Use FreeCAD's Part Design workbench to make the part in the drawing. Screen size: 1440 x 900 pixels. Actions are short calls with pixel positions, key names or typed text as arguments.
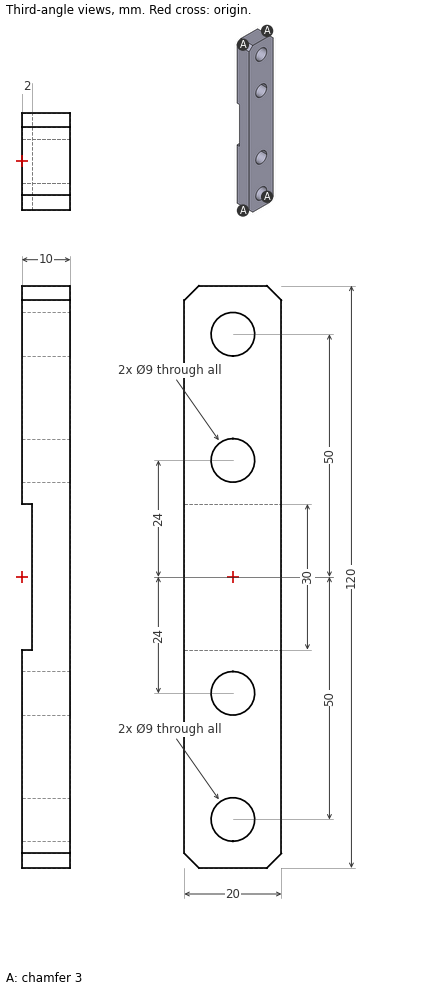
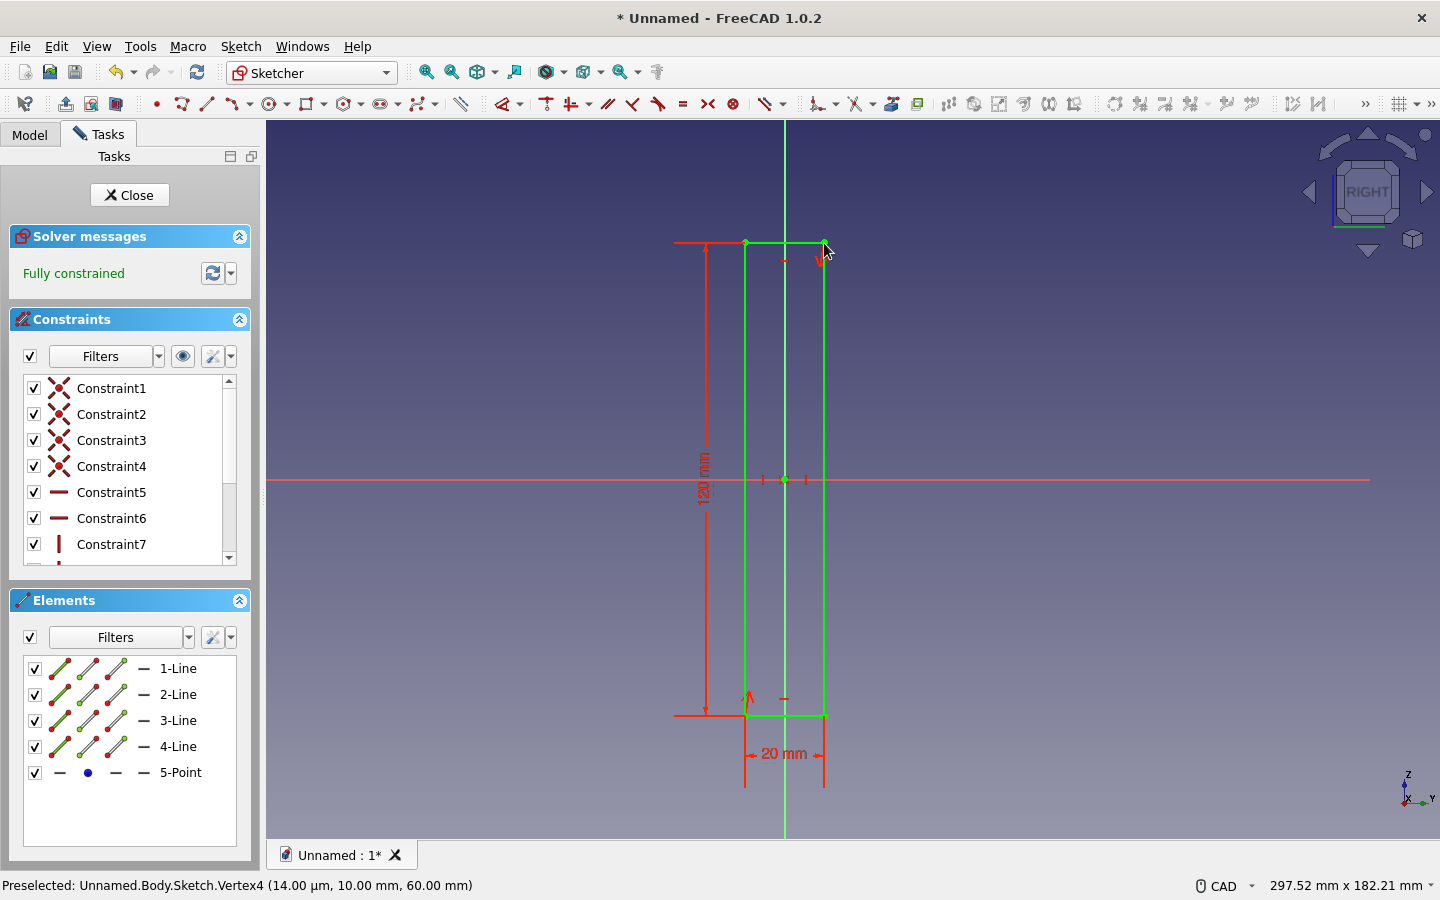
click(130, 195)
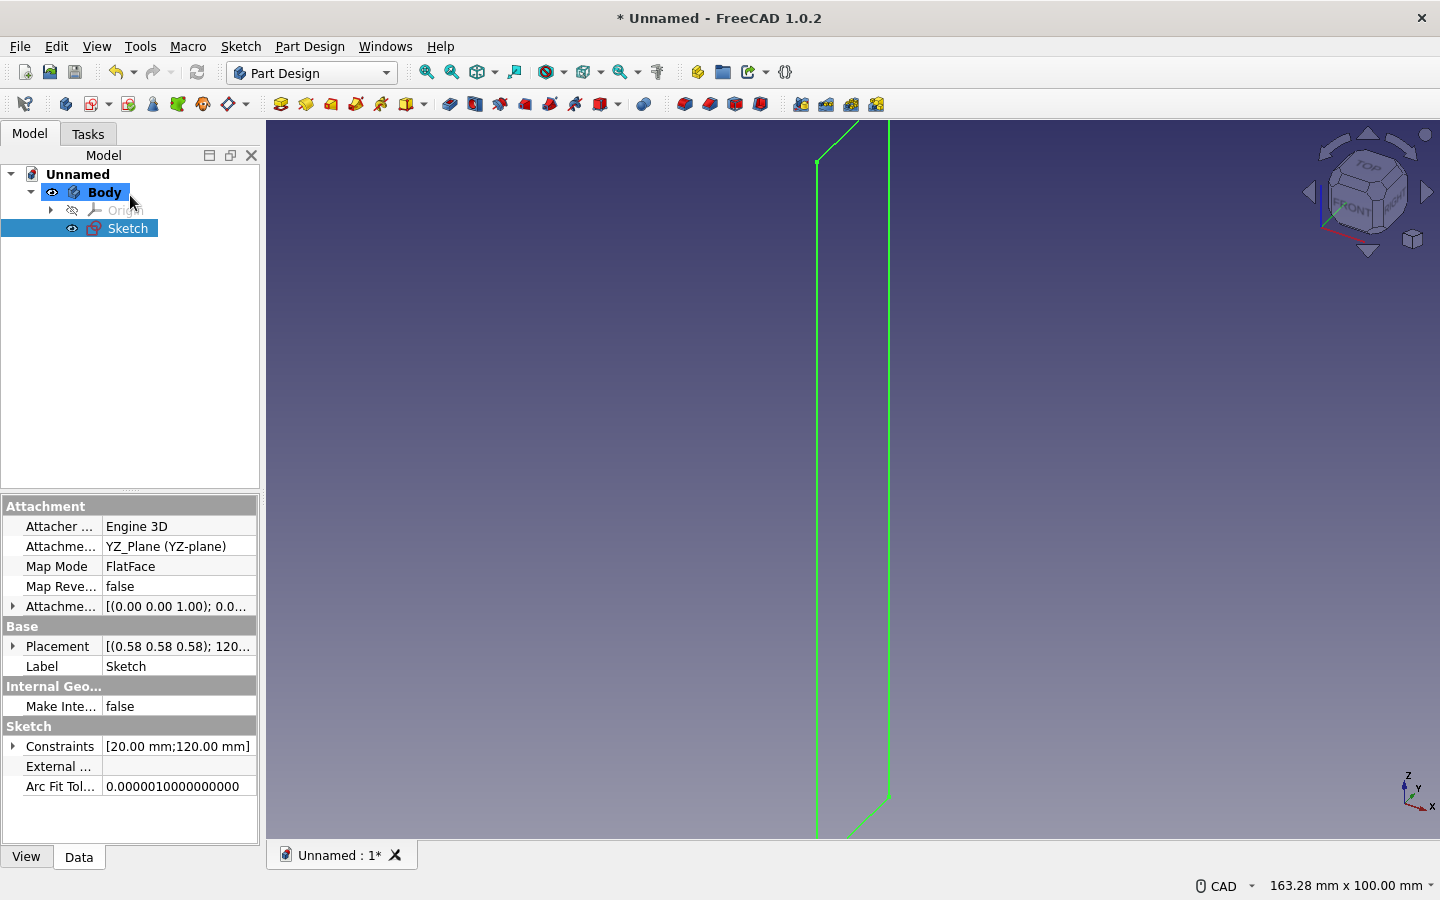
click(281, 104)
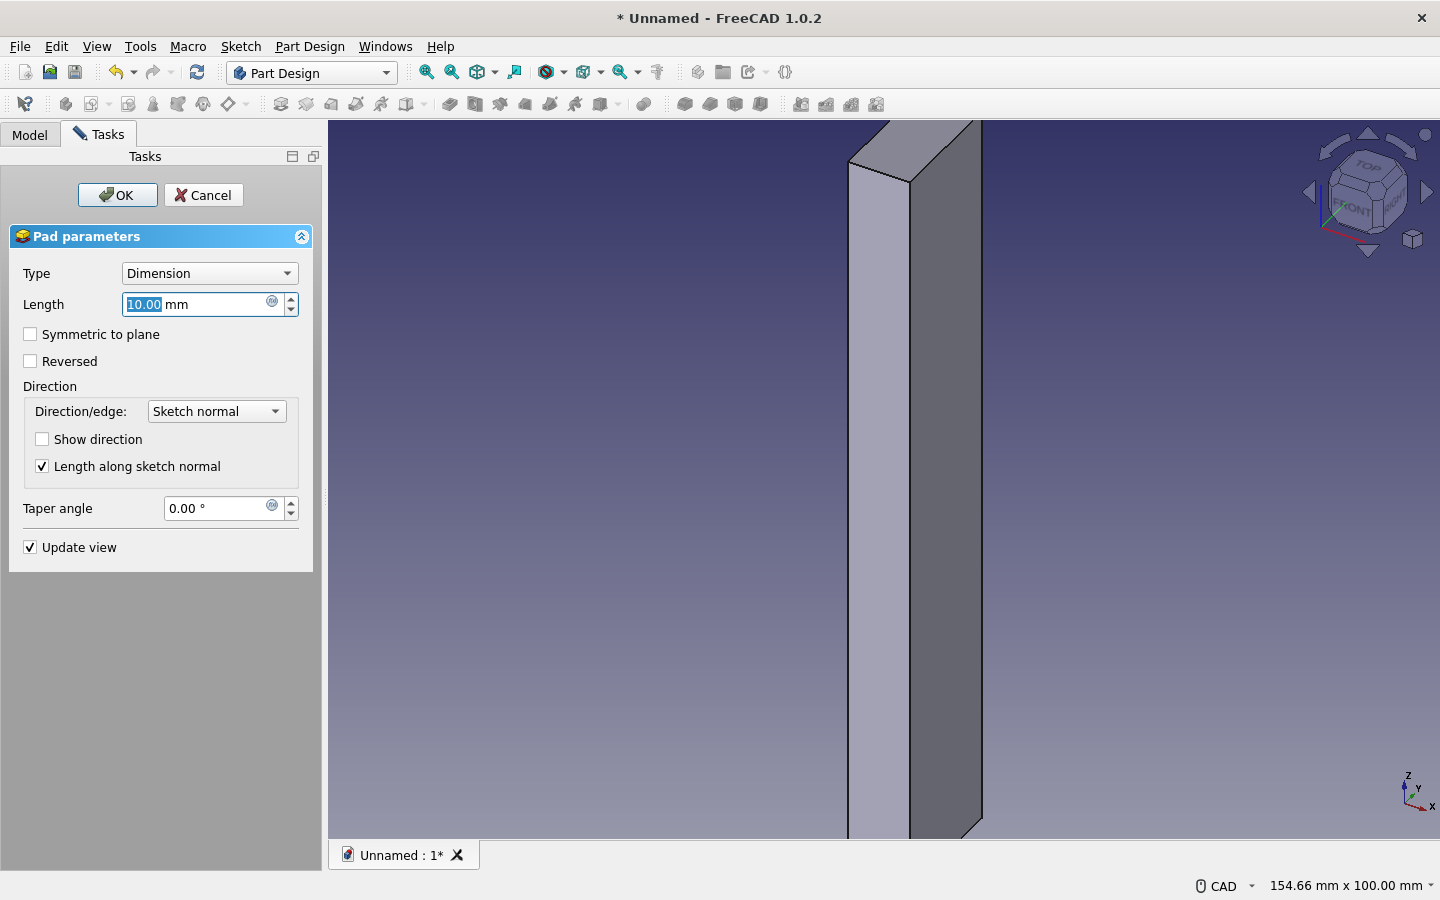
text(10)
key(Tab)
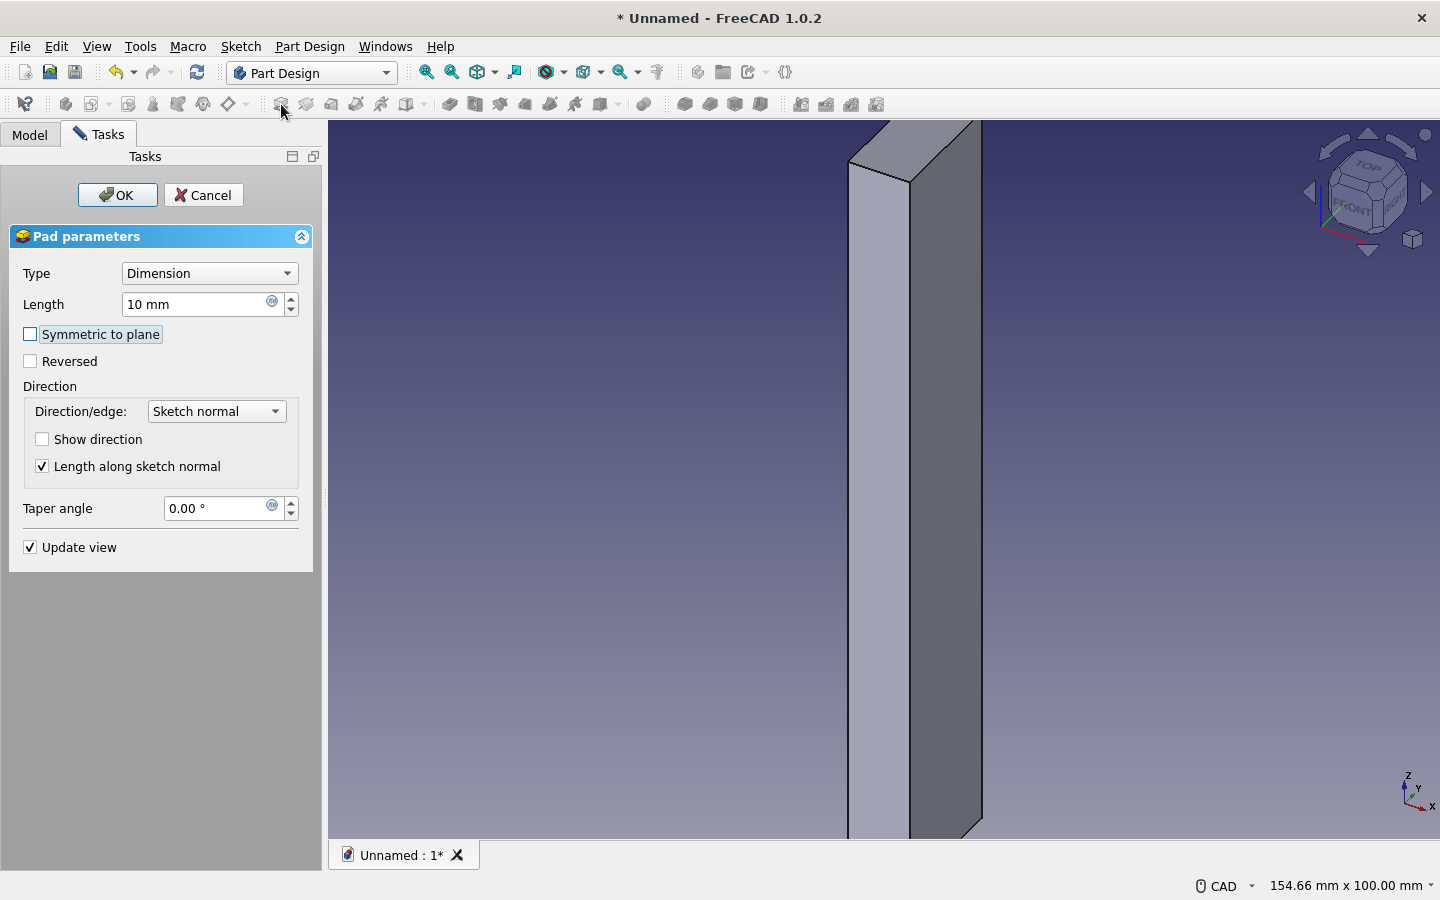
click(118, 195)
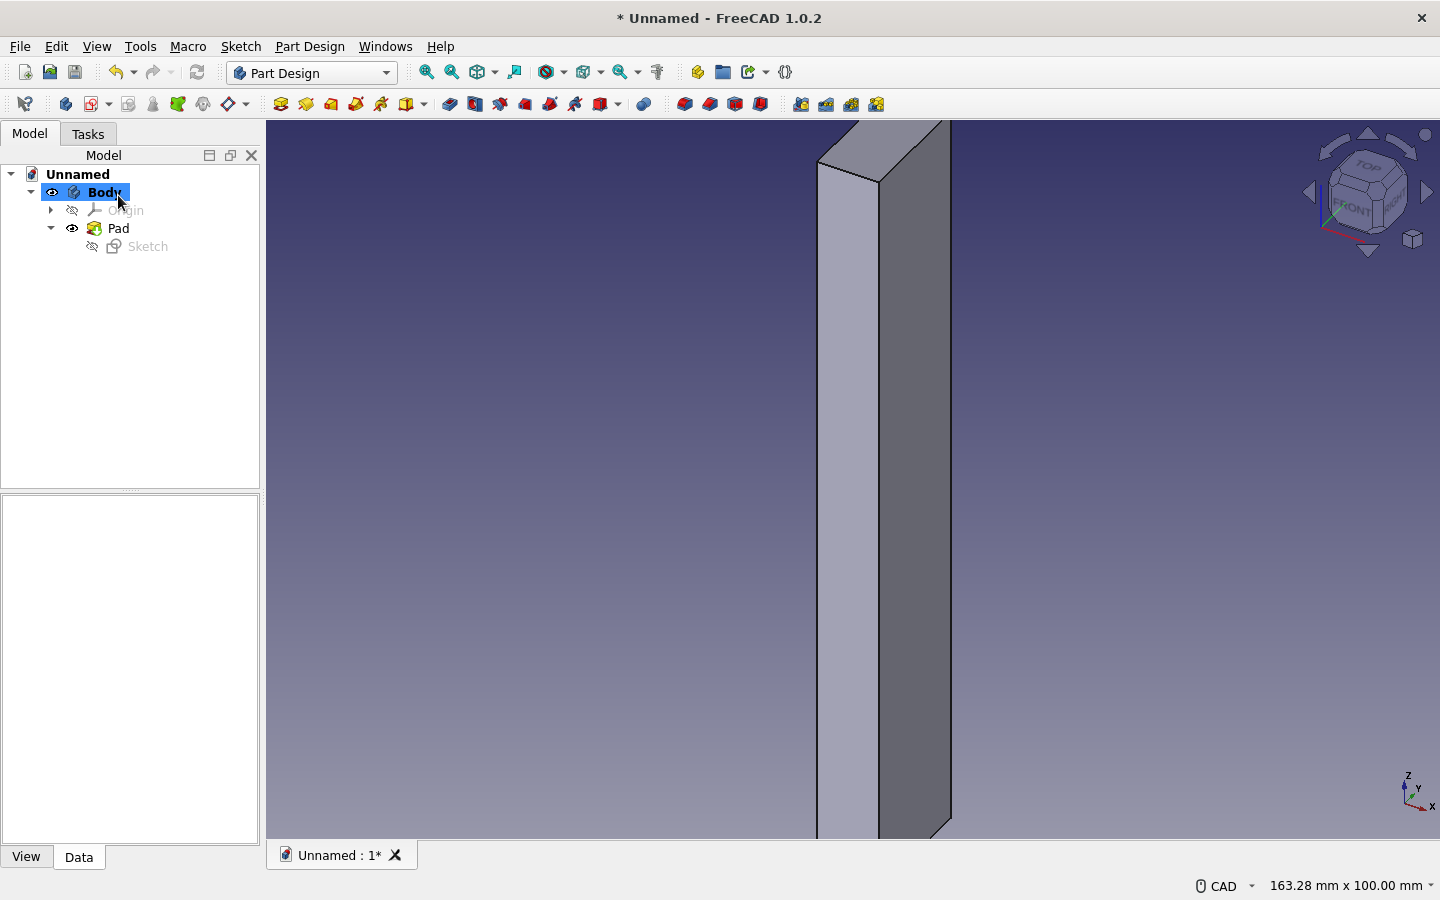
key(v)
key(f)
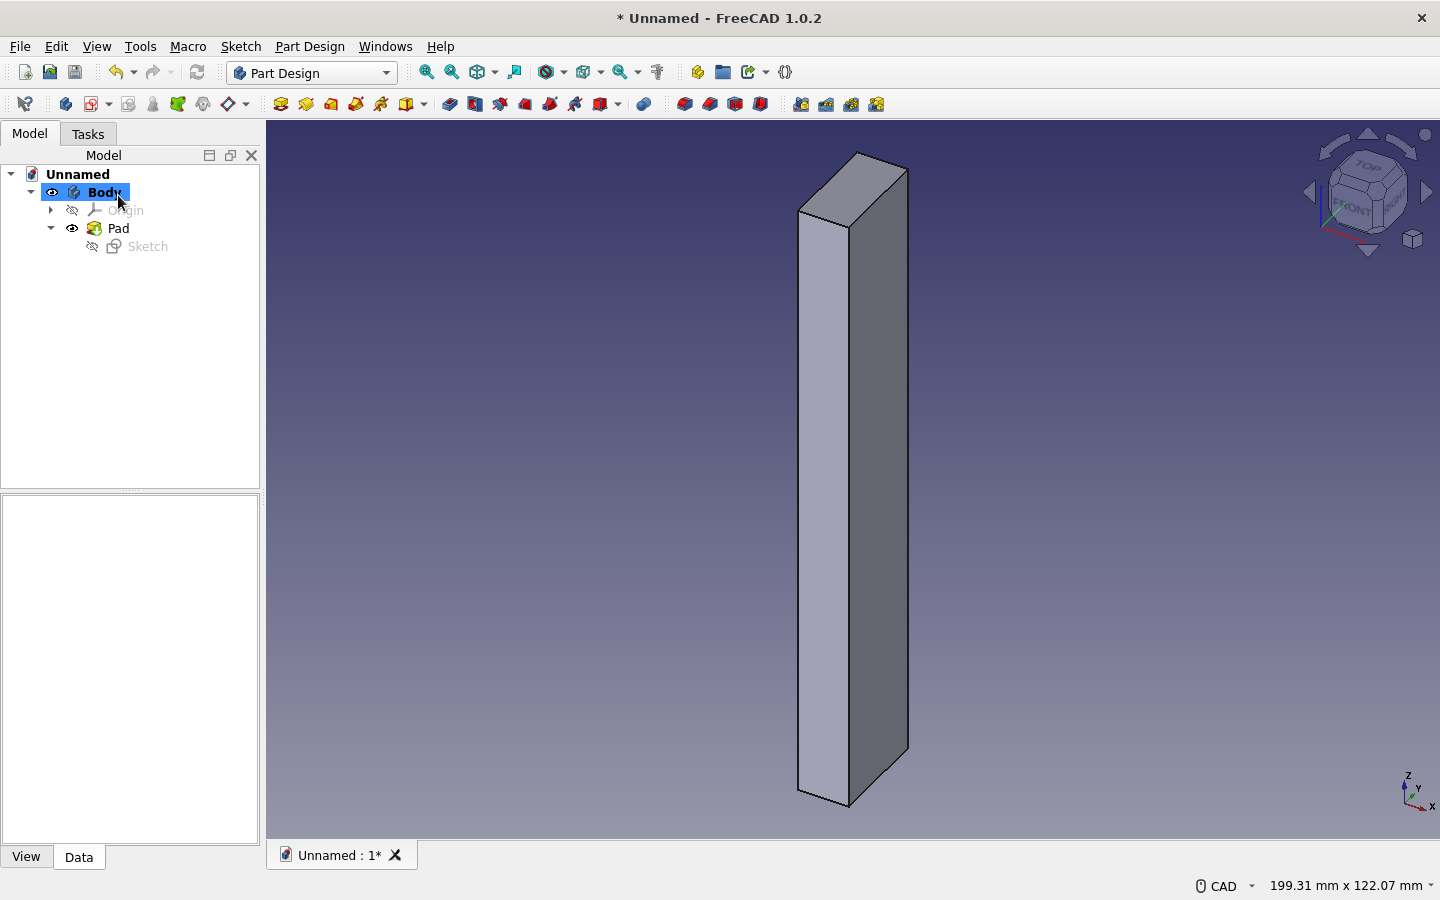
click(879, 652)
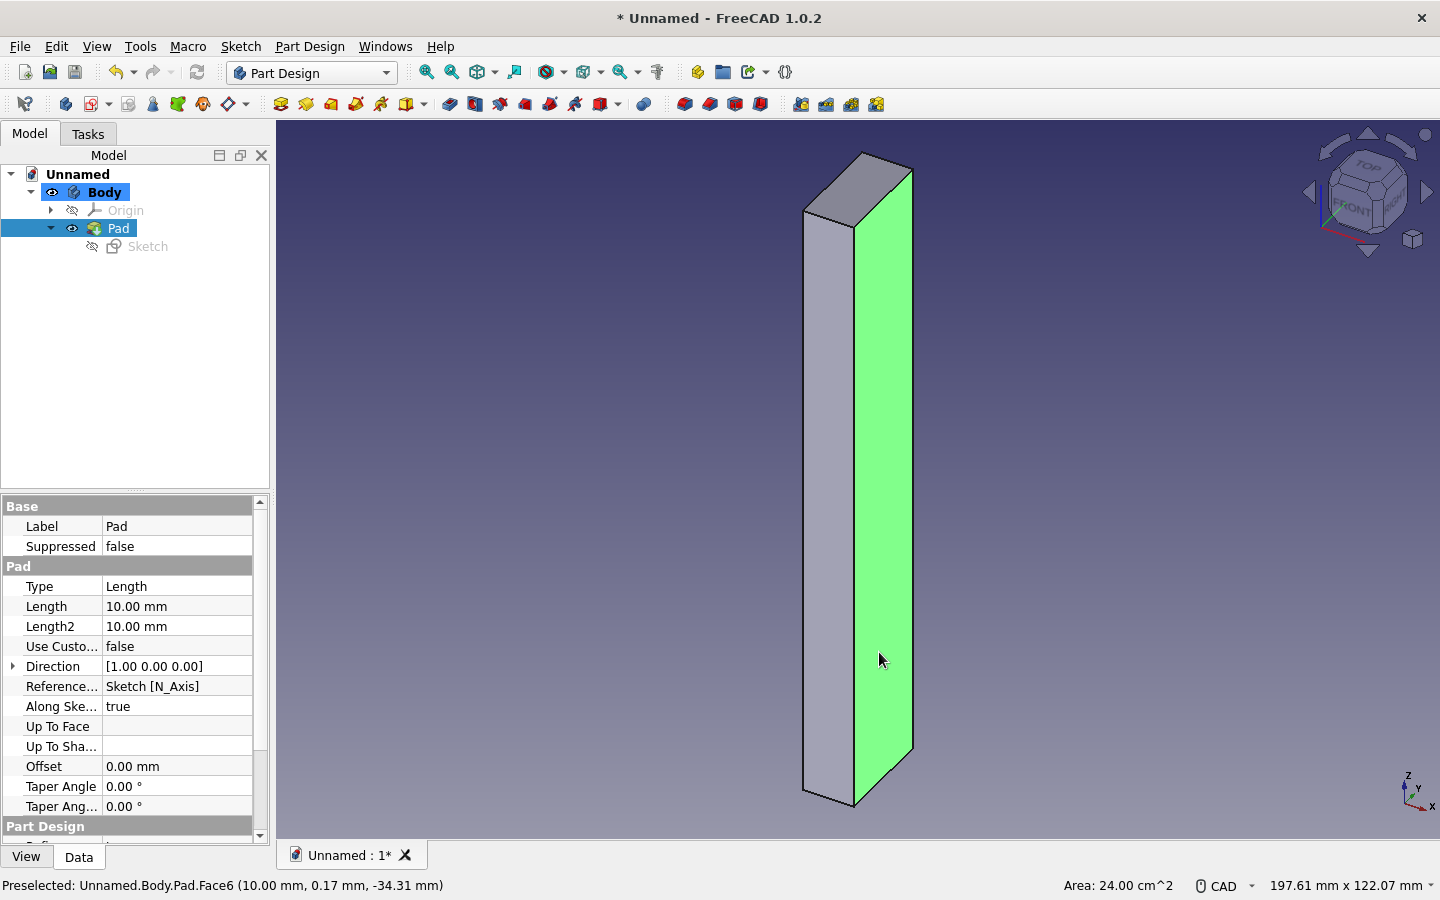
click(90, 104)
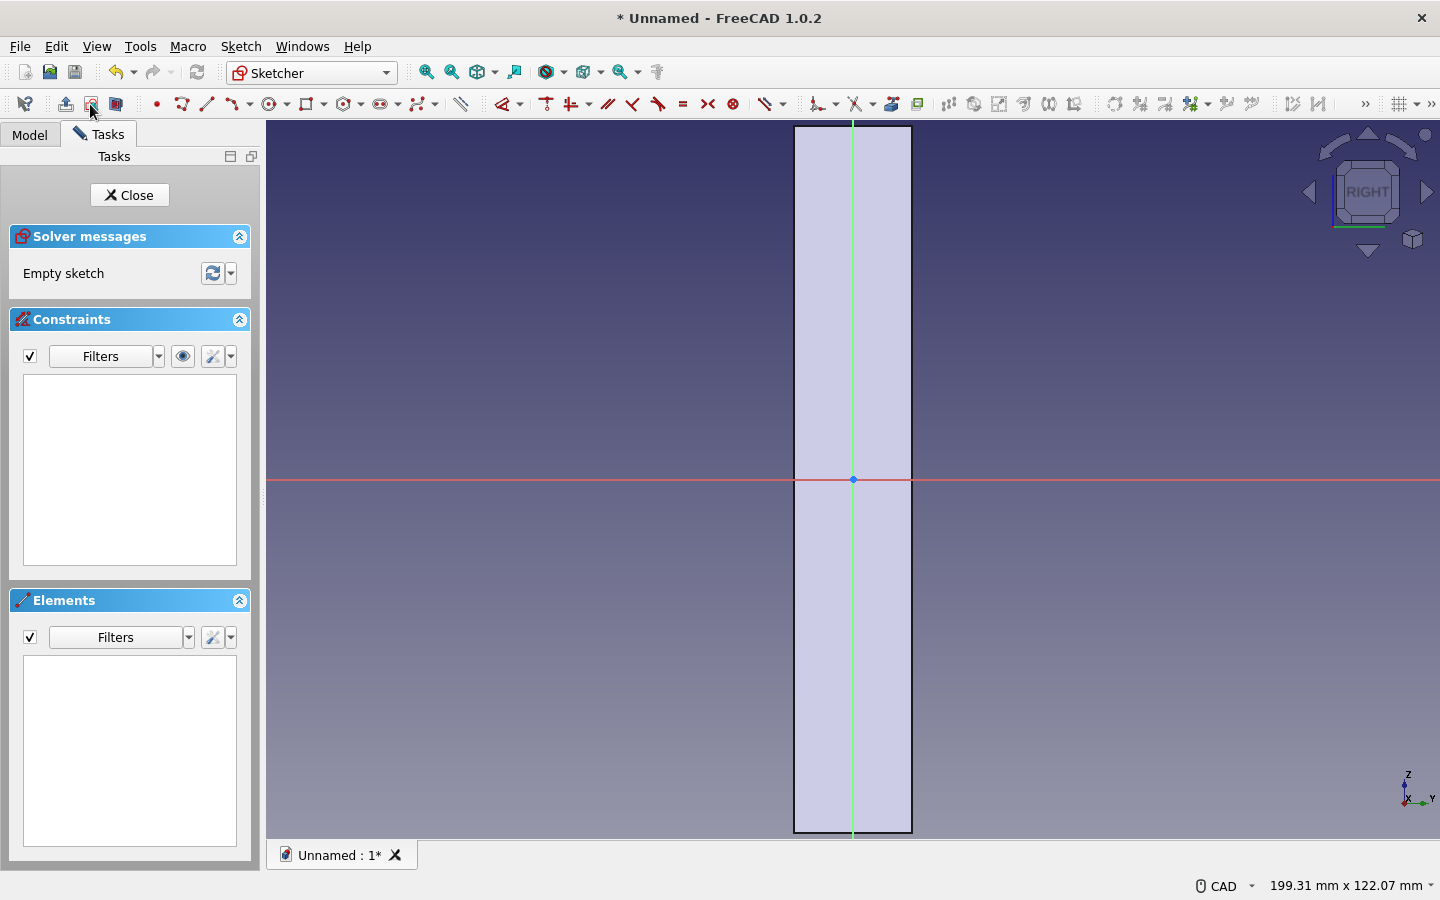
scroll(992, 480, up, 2)